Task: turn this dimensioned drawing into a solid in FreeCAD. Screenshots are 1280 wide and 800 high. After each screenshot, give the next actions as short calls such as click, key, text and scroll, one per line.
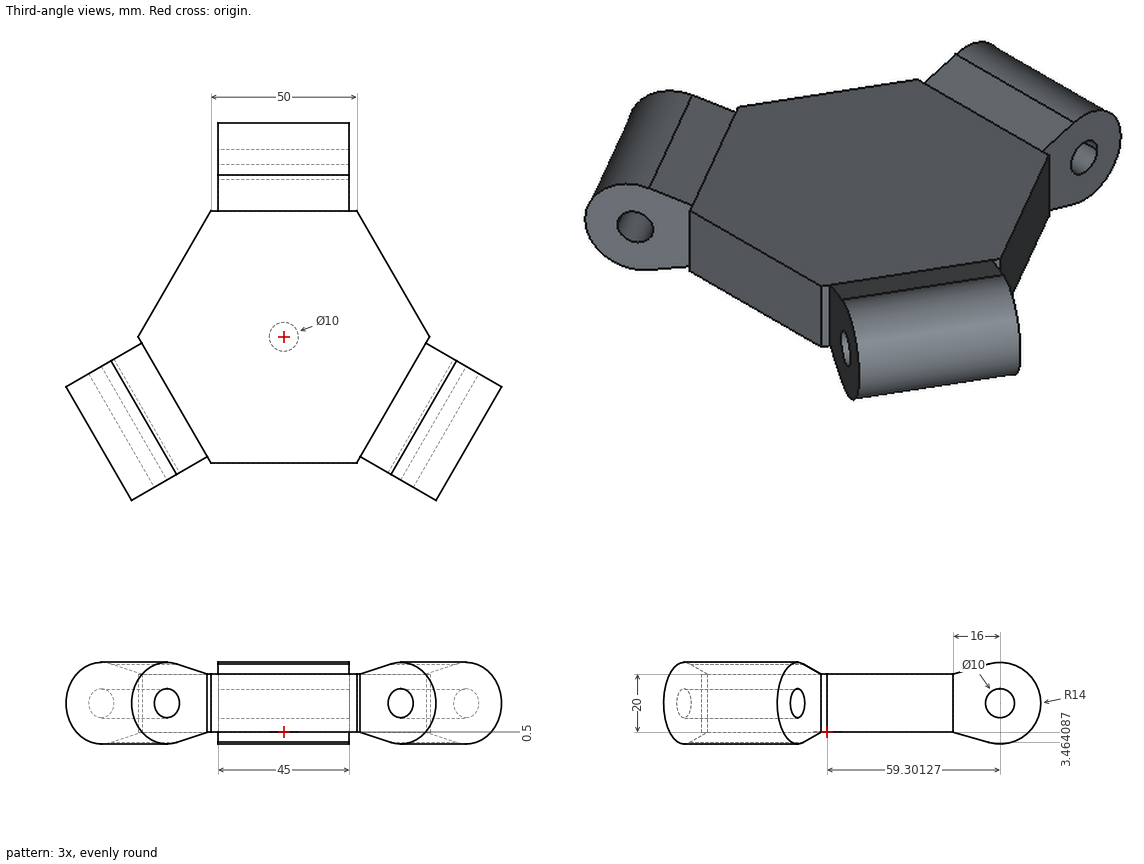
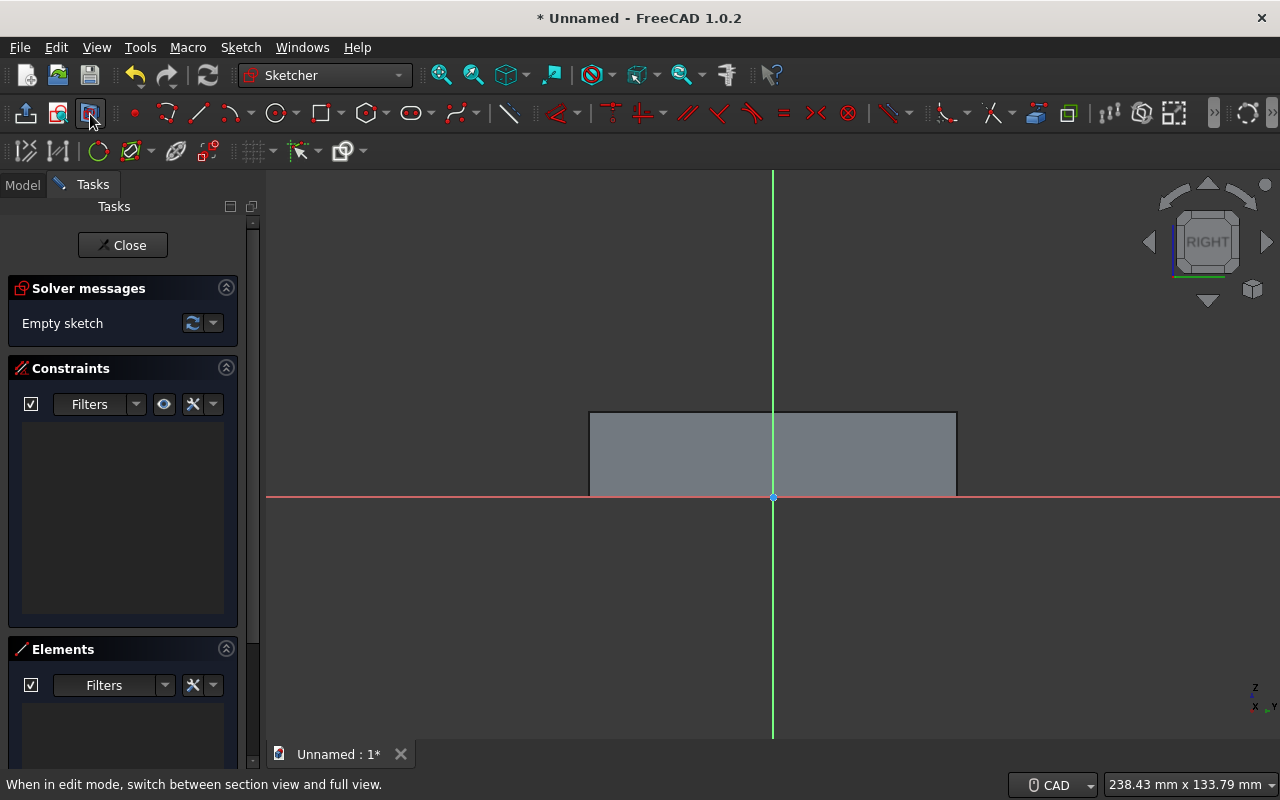
scroll(1115, 454, up, 3)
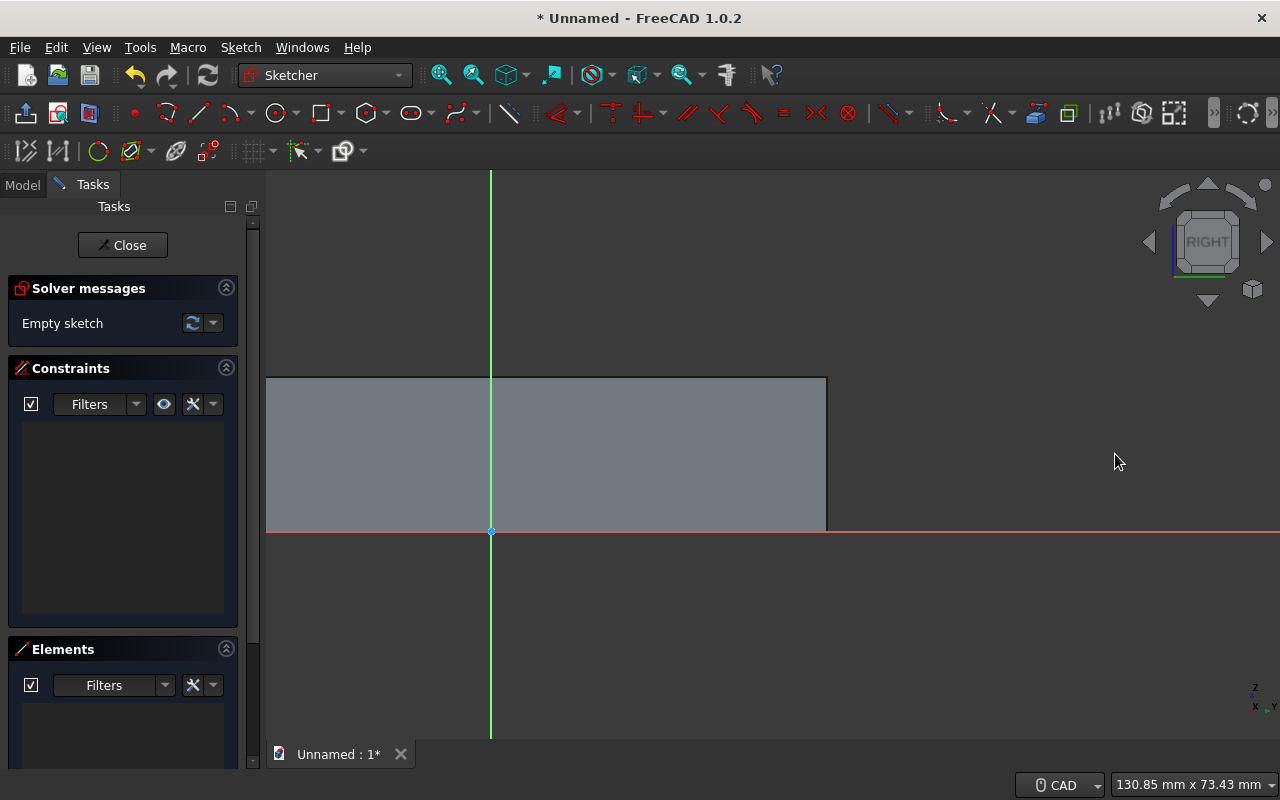
click(168, 114)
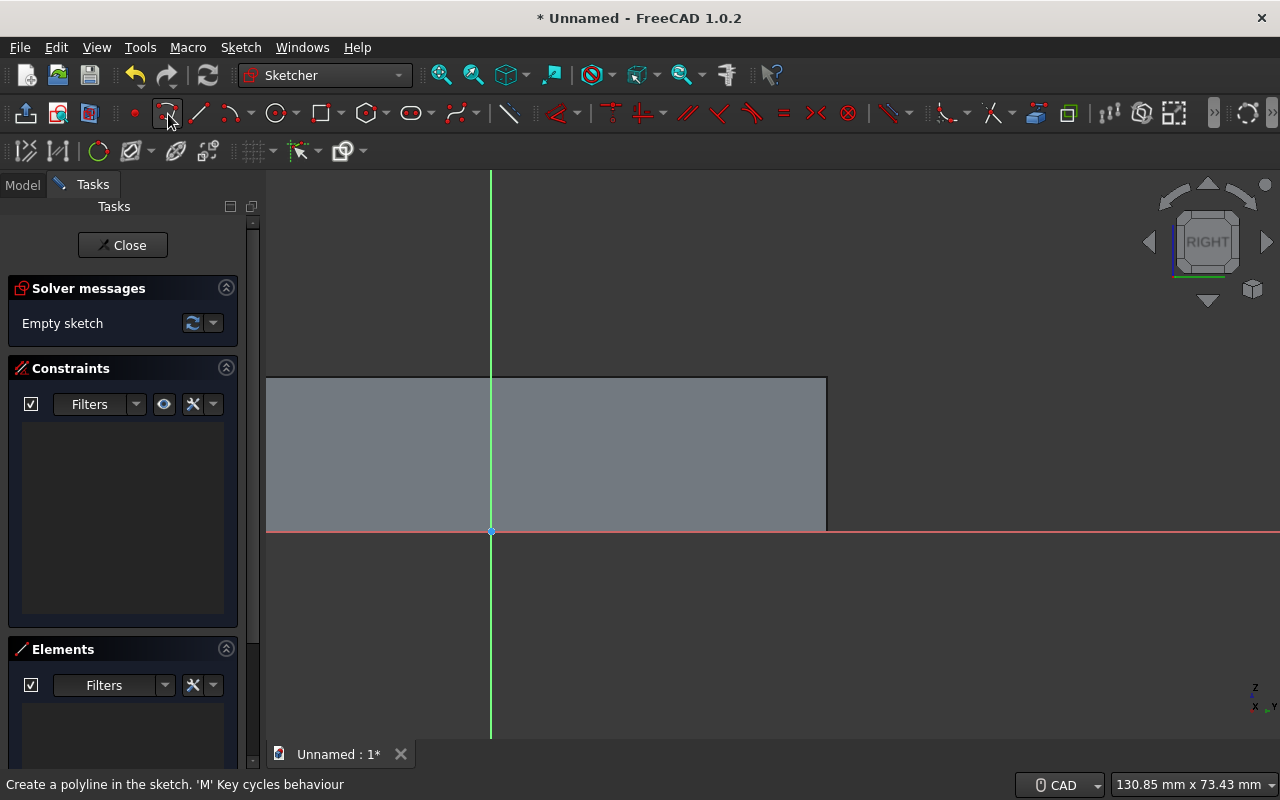
click(921, 350)
click(827, 377)
click(827, 532)
click(921, 559)
right_click(921, 559)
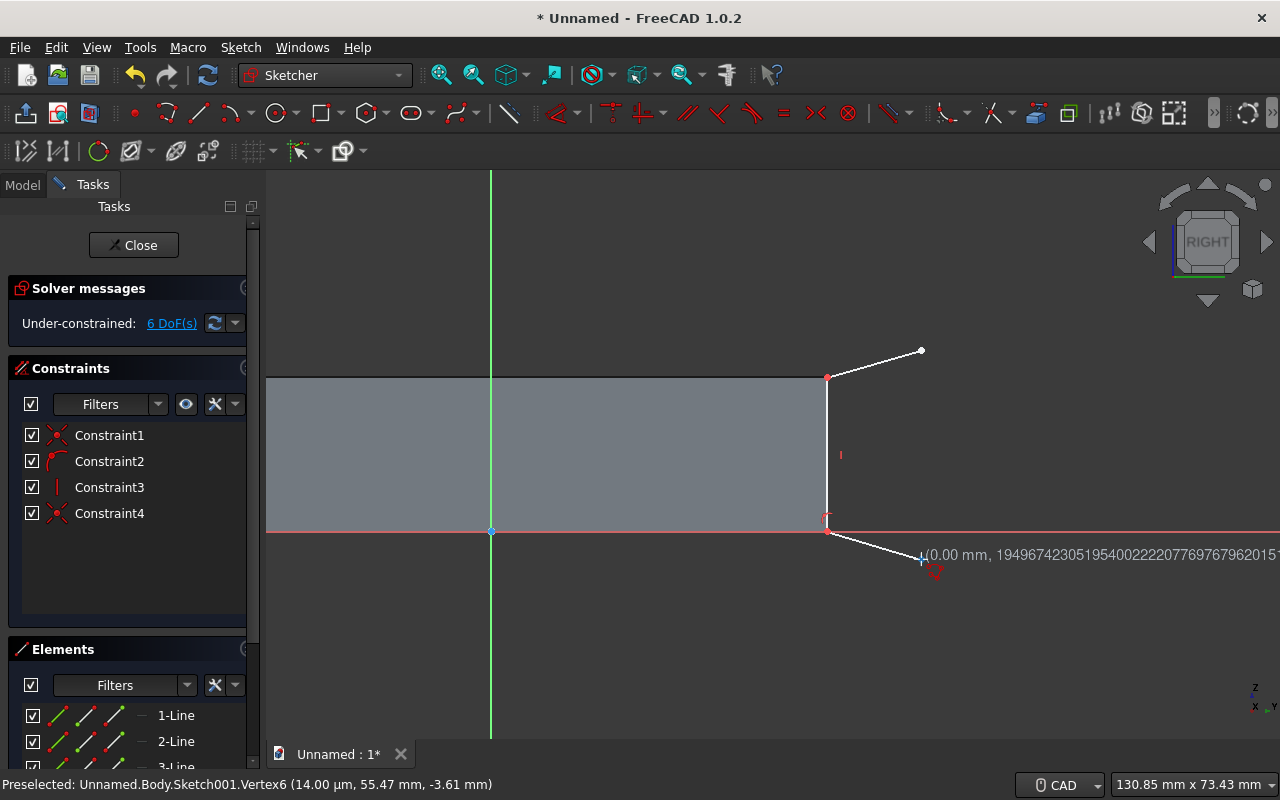
click(254, 114)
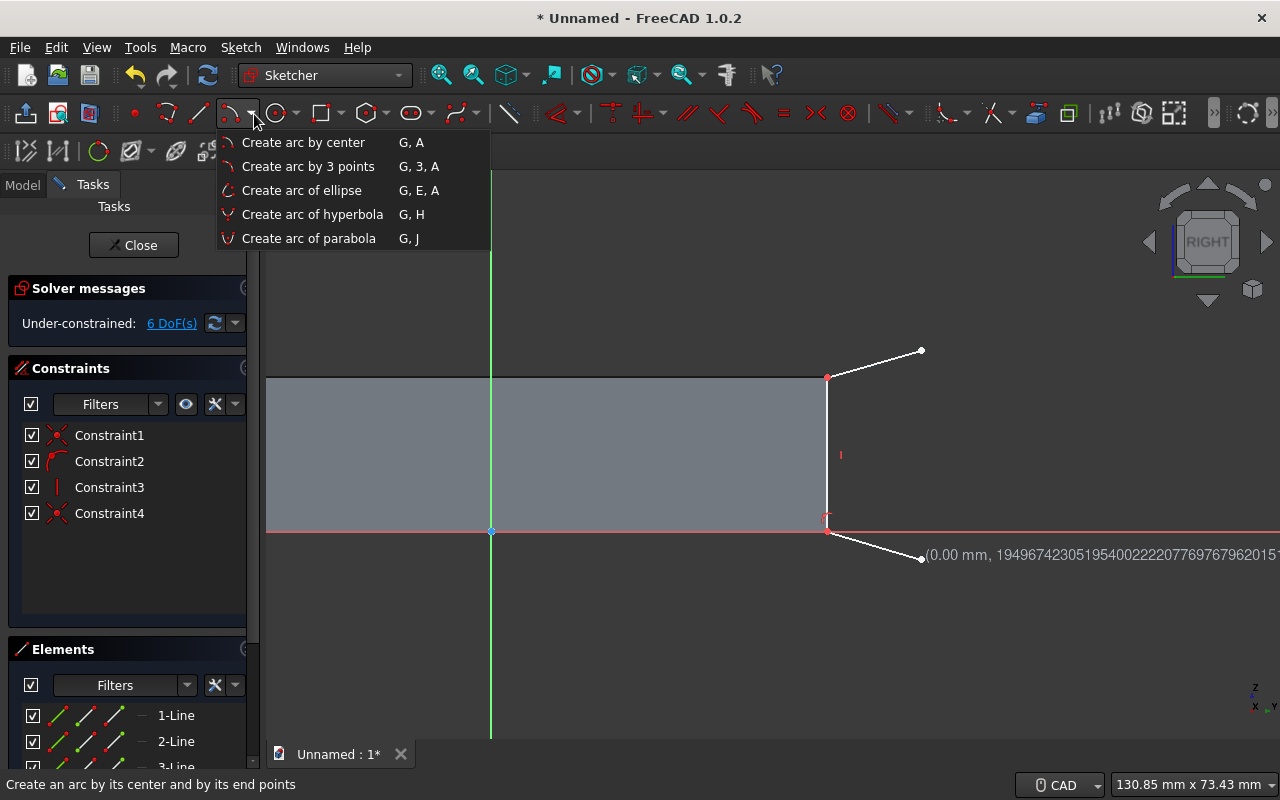
click(354, 166)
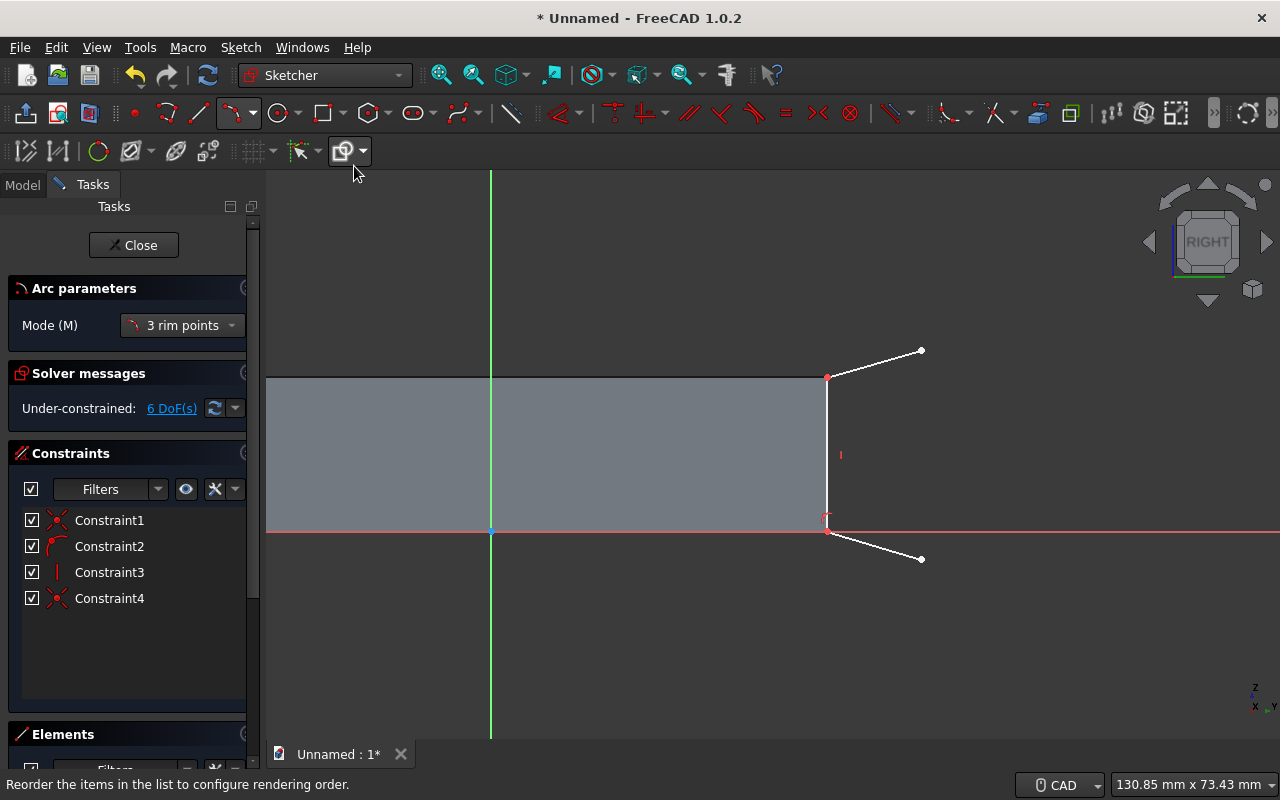
click(921, 560)
click(921, 351)
click(1059, 454)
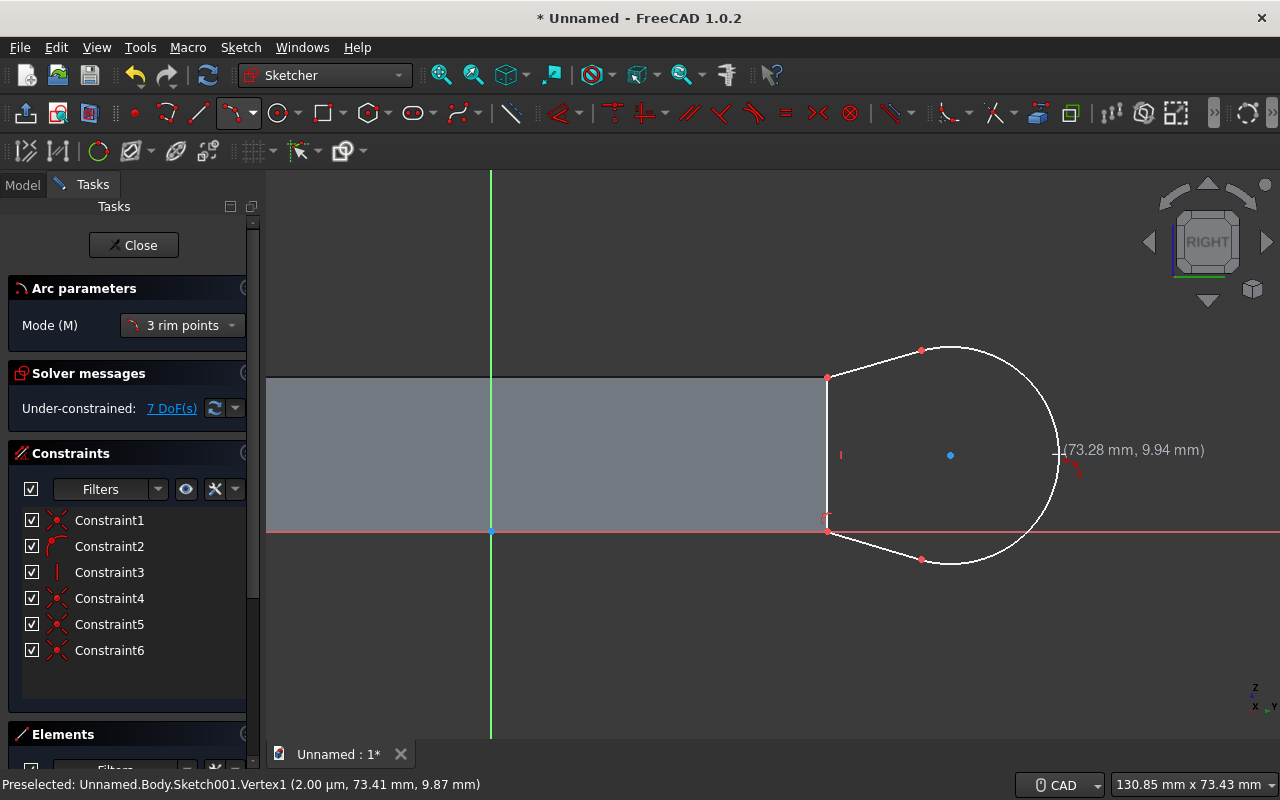
click(278, 114)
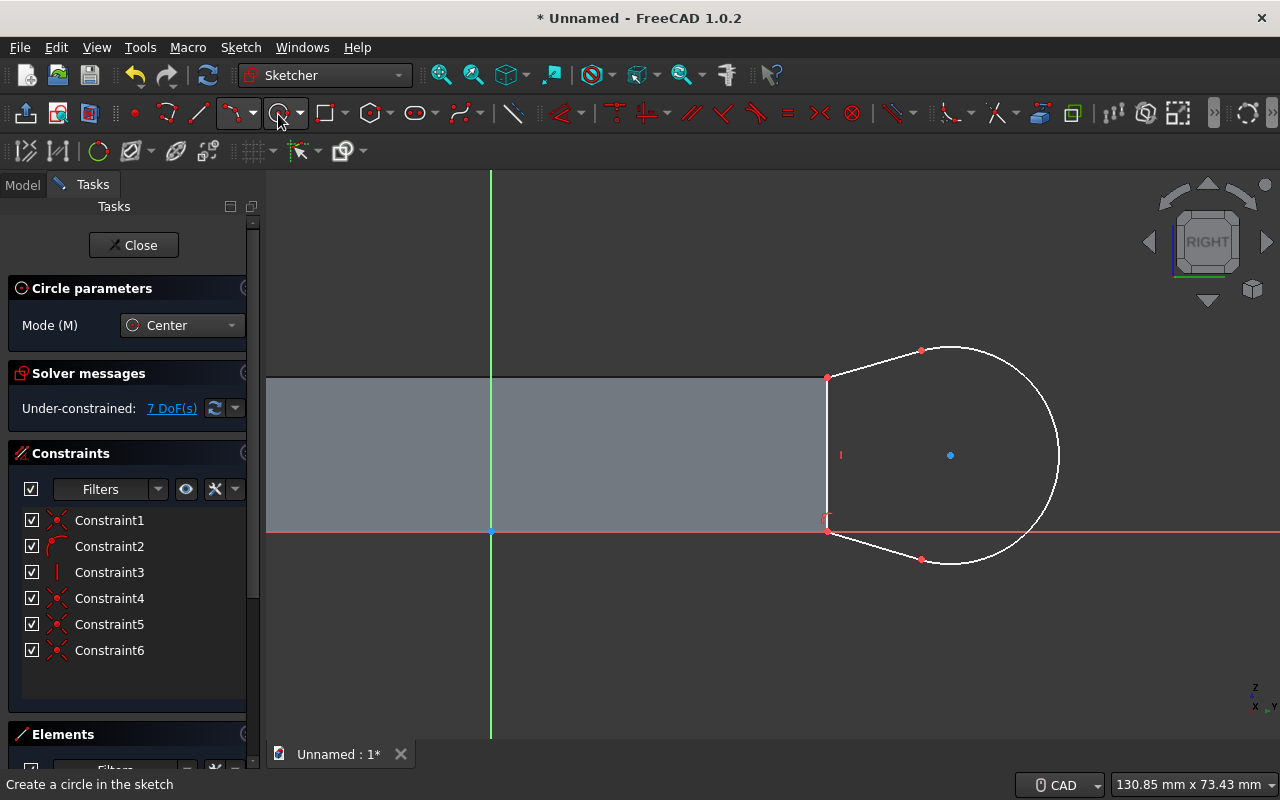
click(951, 454)
move(978, 427)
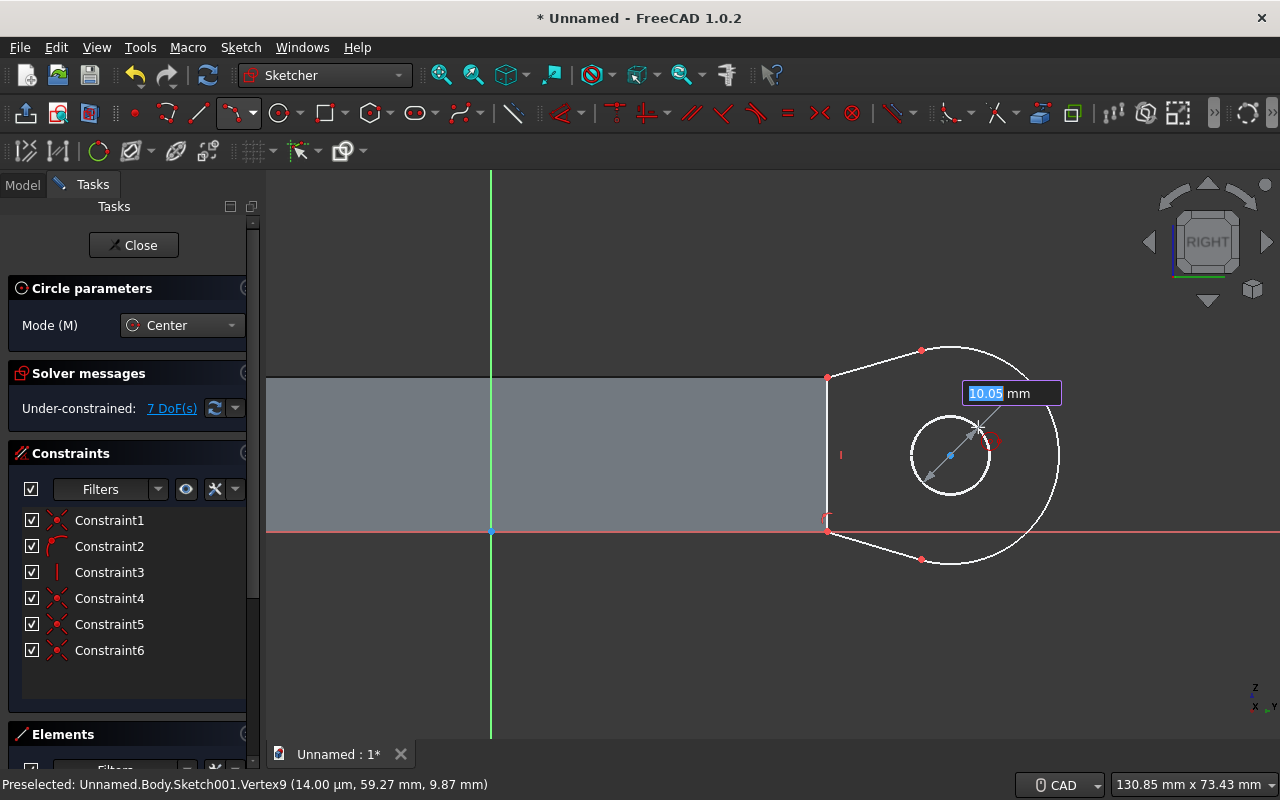
text(10)
key(Return)
key(Escape)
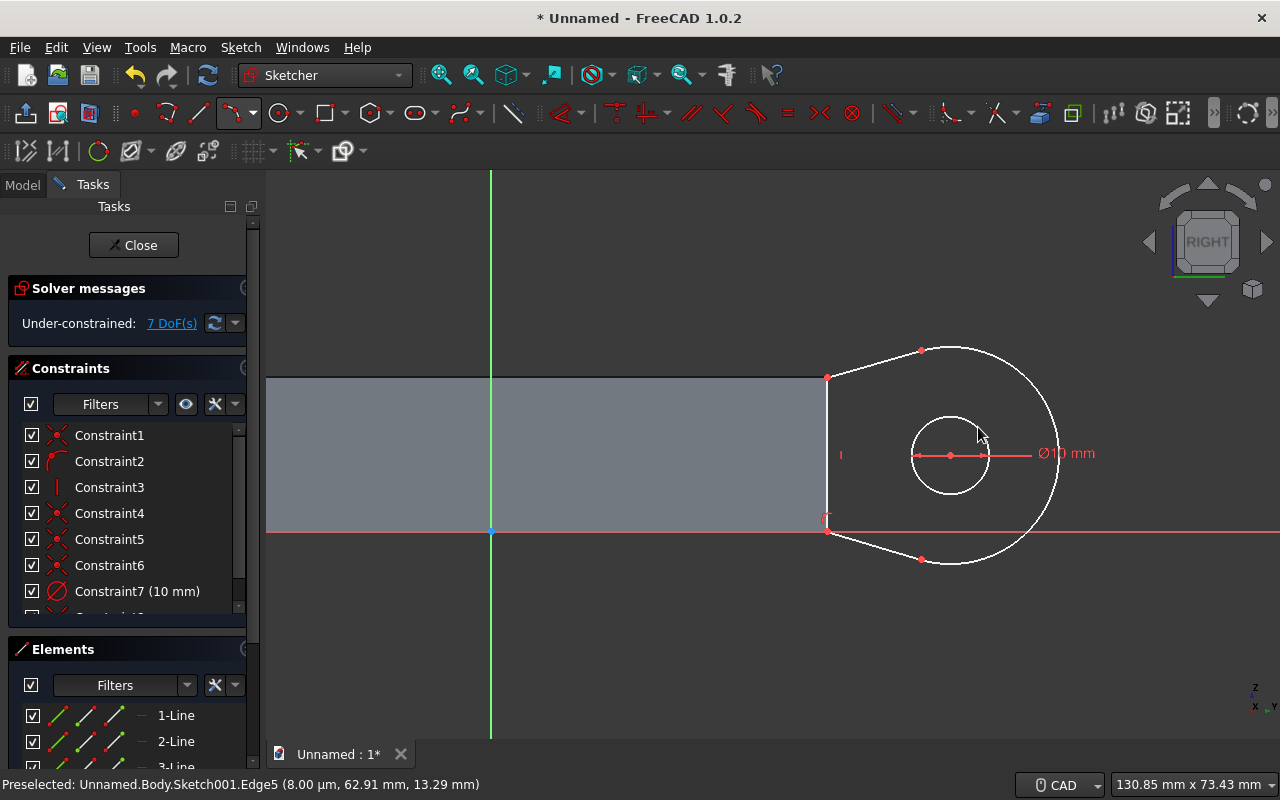
click(893, 359)